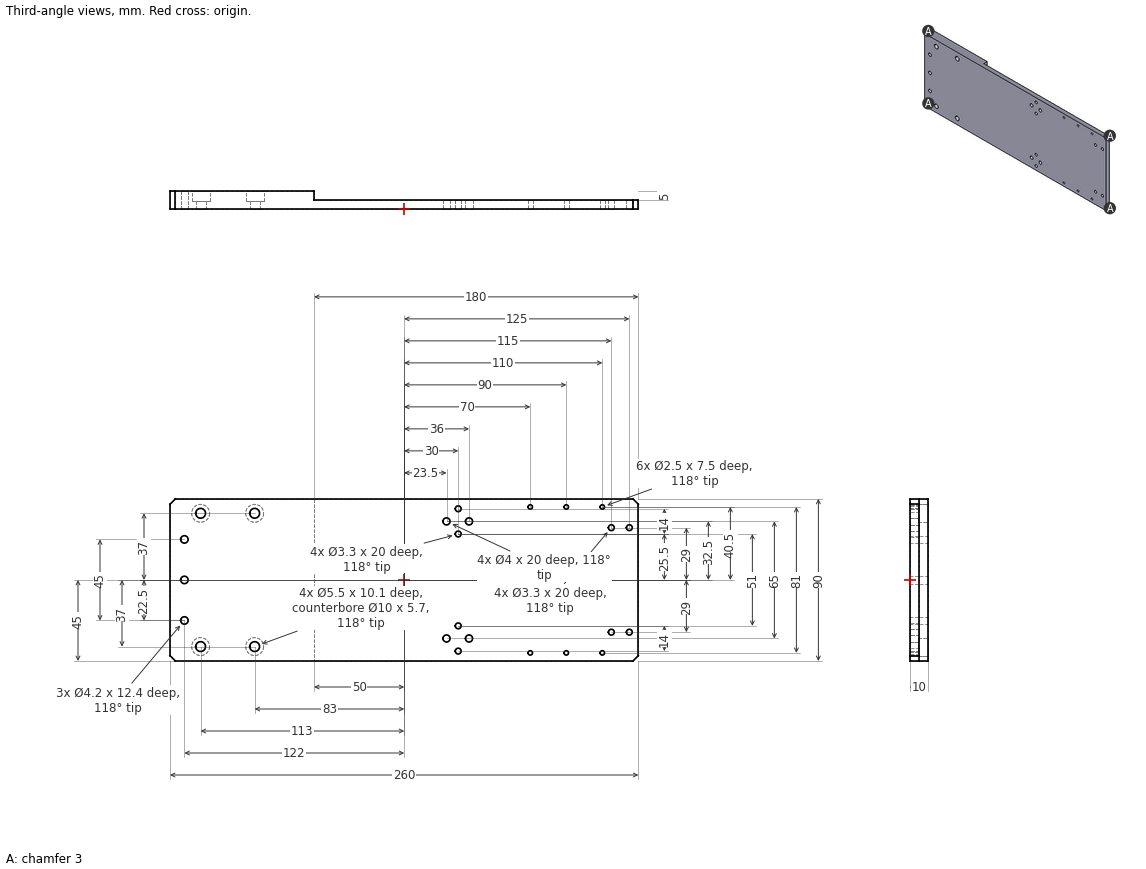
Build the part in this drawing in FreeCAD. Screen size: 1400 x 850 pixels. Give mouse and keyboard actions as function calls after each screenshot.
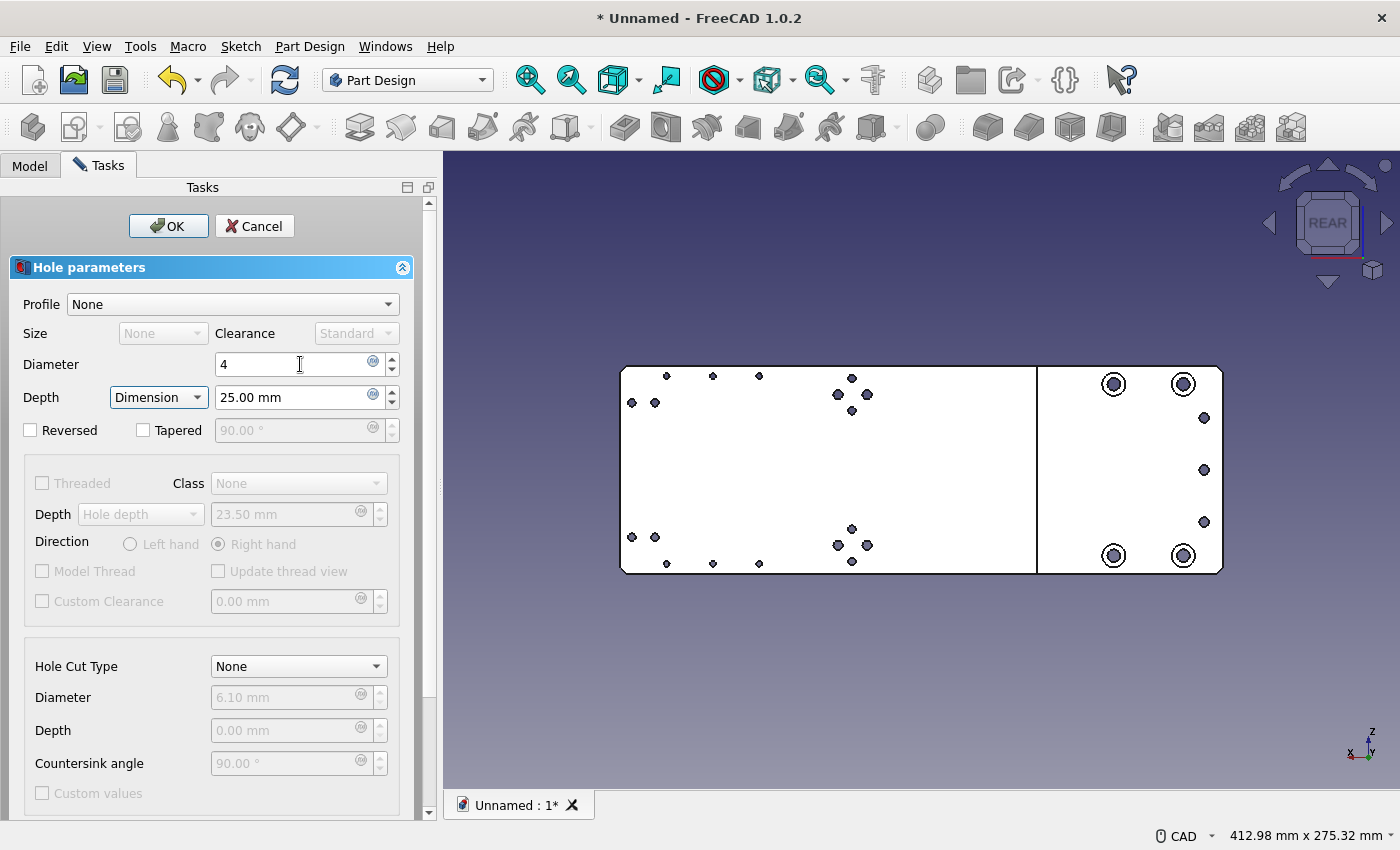
triple_click(300, 398)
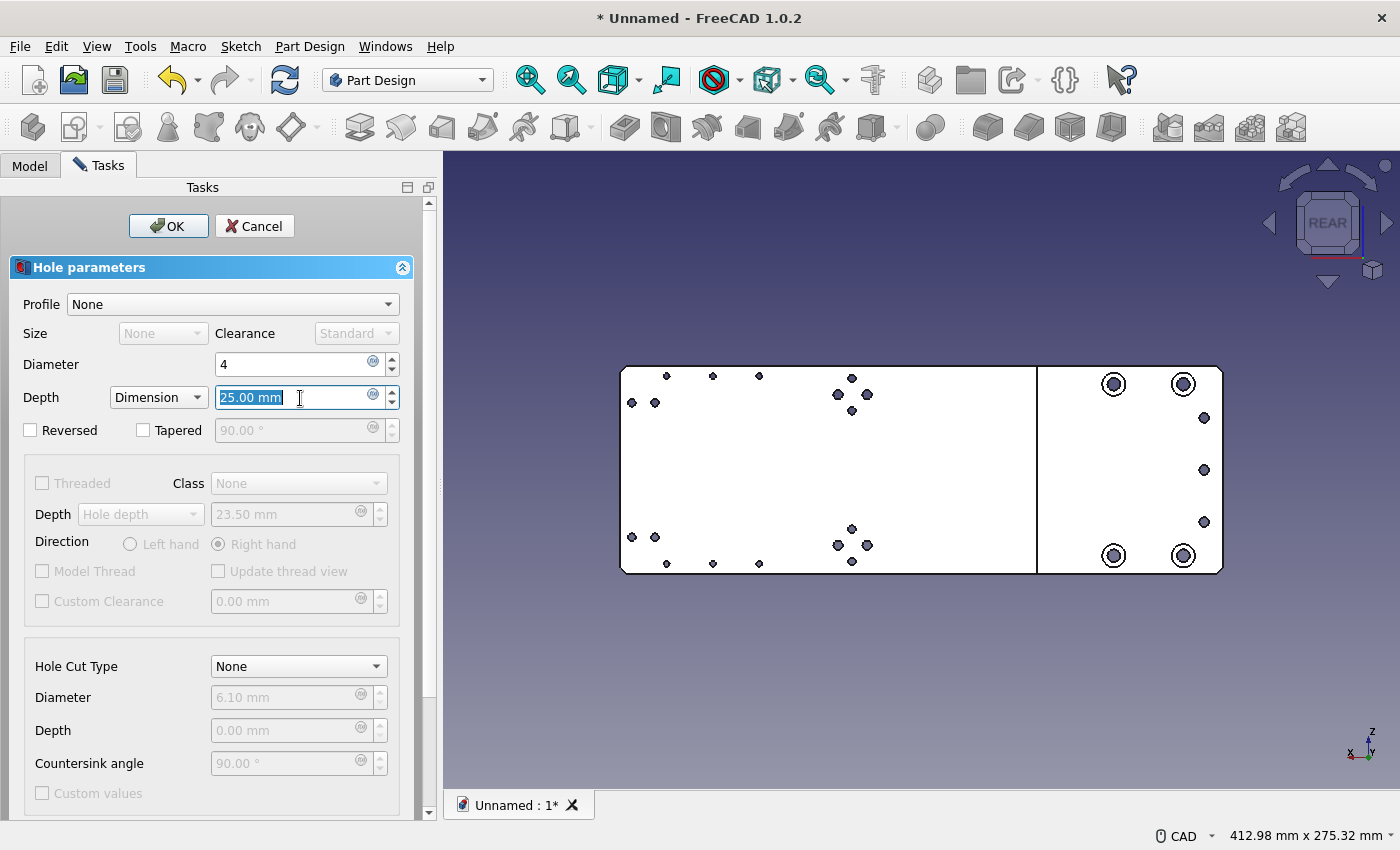
text(20)
key(Tab)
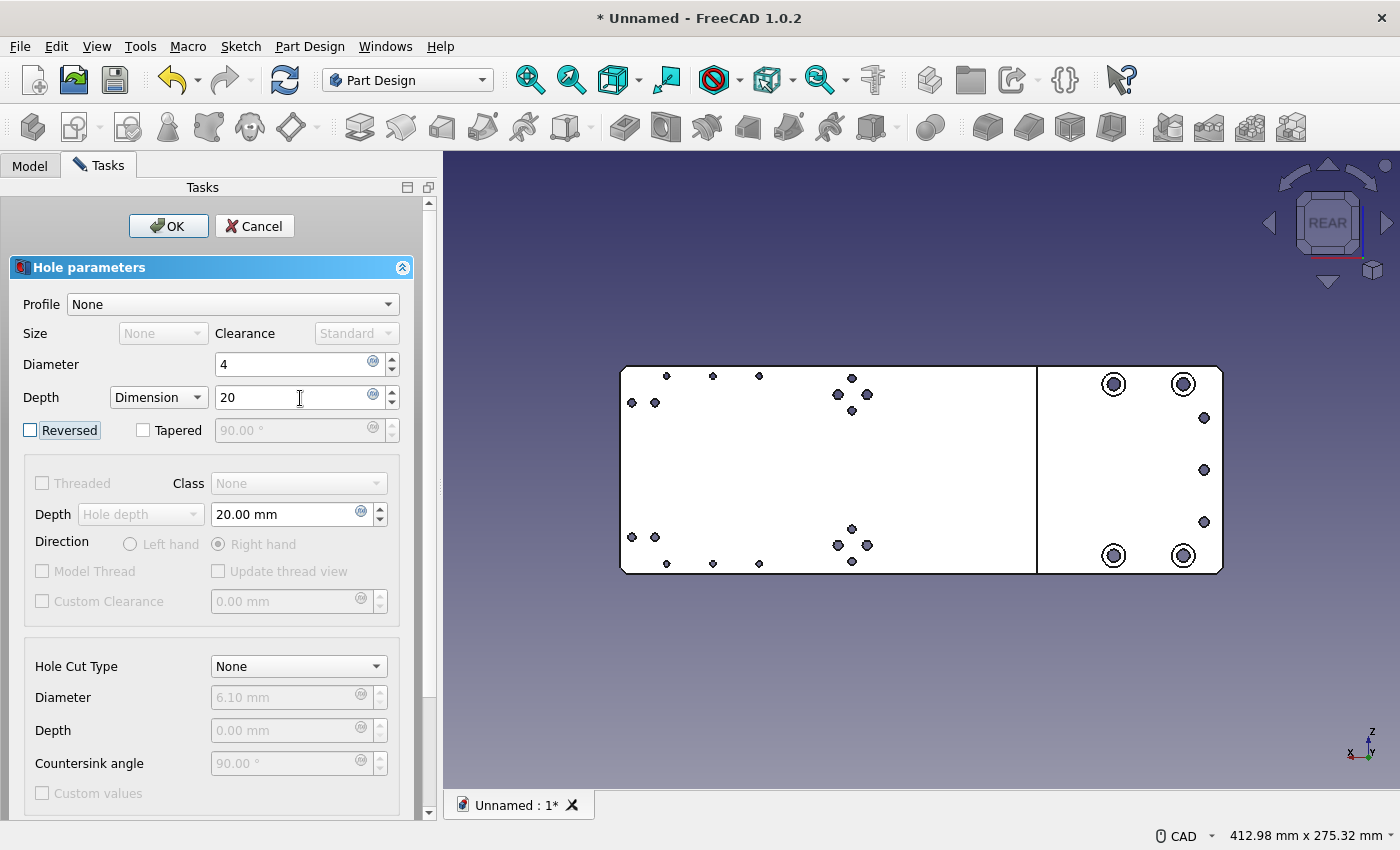
click(169, 226)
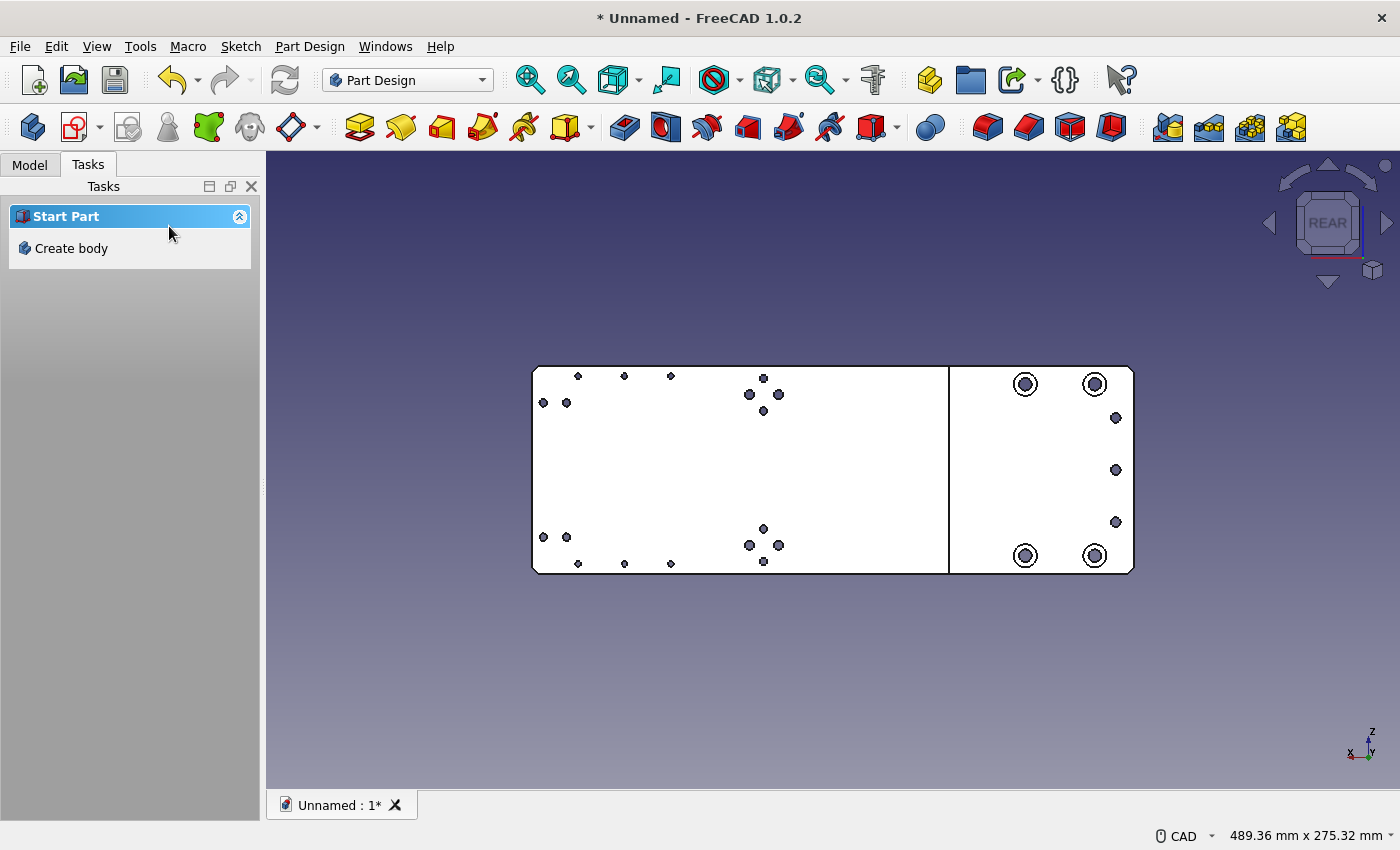
key(0)